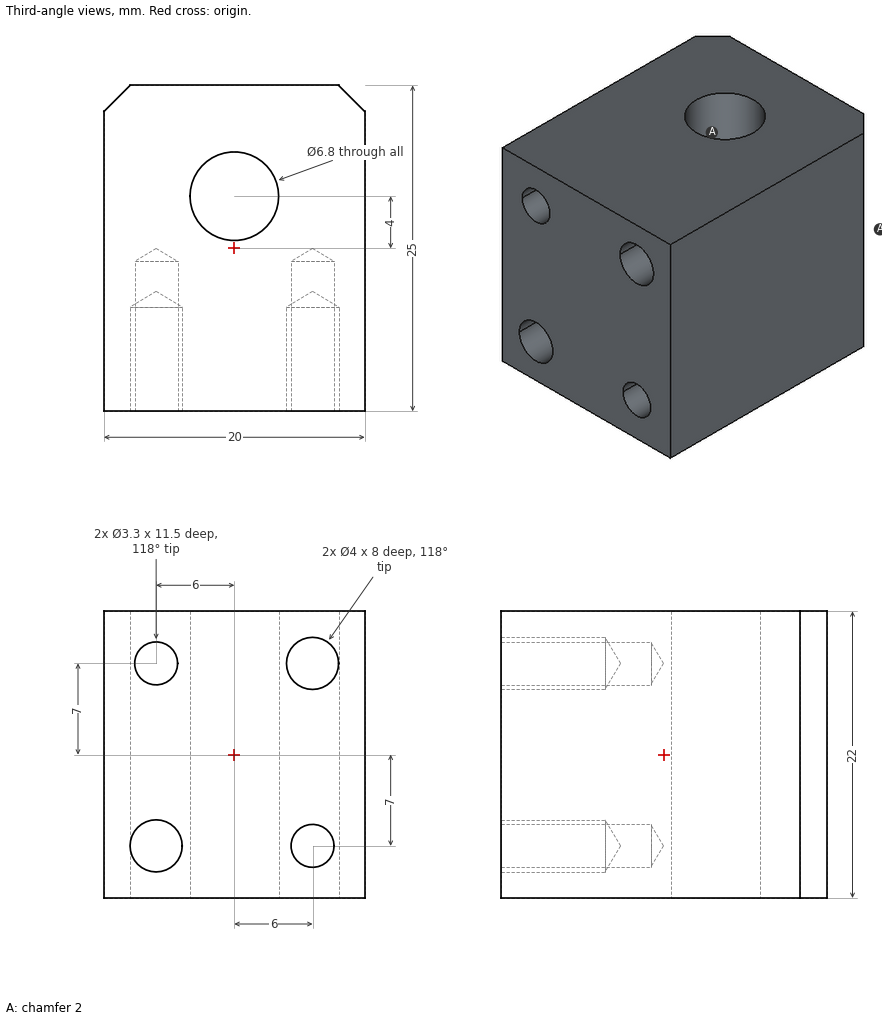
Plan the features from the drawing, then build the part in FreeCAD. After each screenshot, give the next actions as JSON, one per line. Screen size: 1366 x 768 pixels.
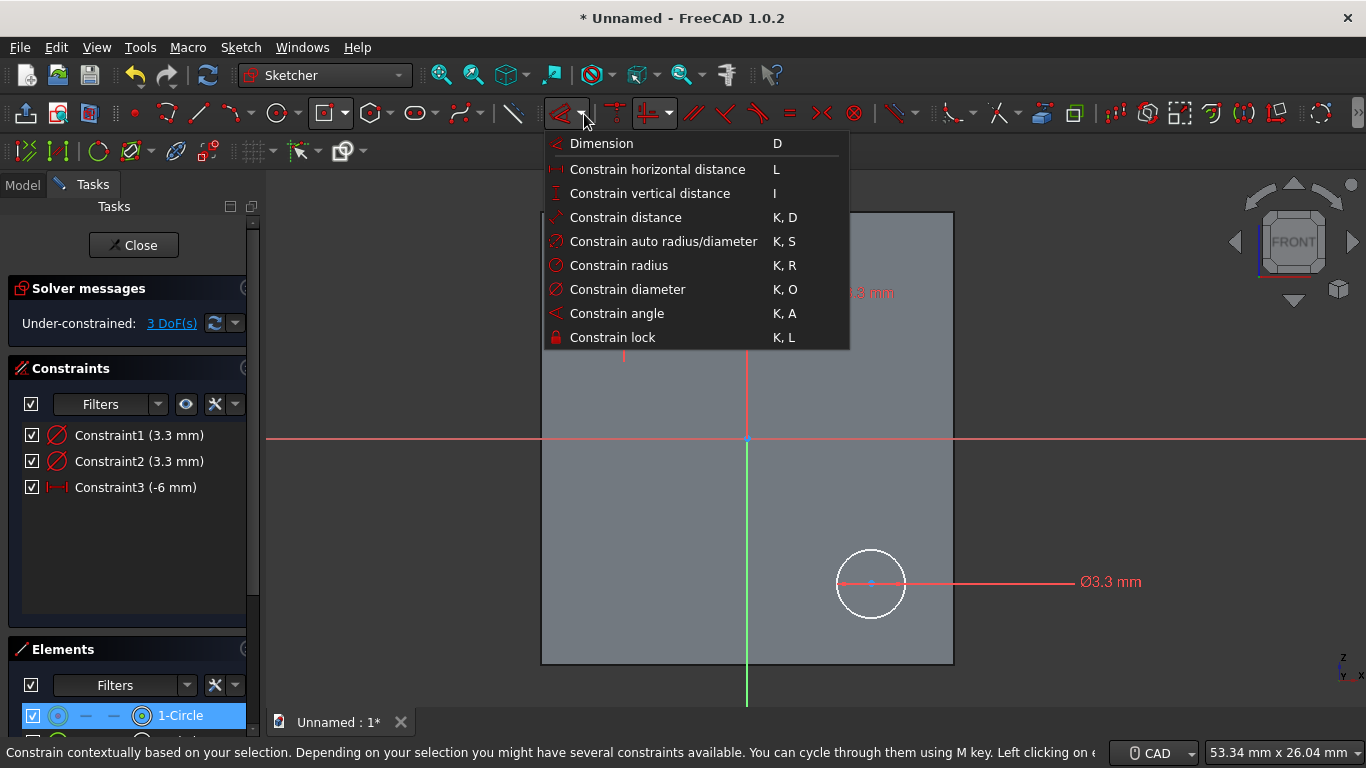
{"action": "left_click", "coordinate": [697, 193]}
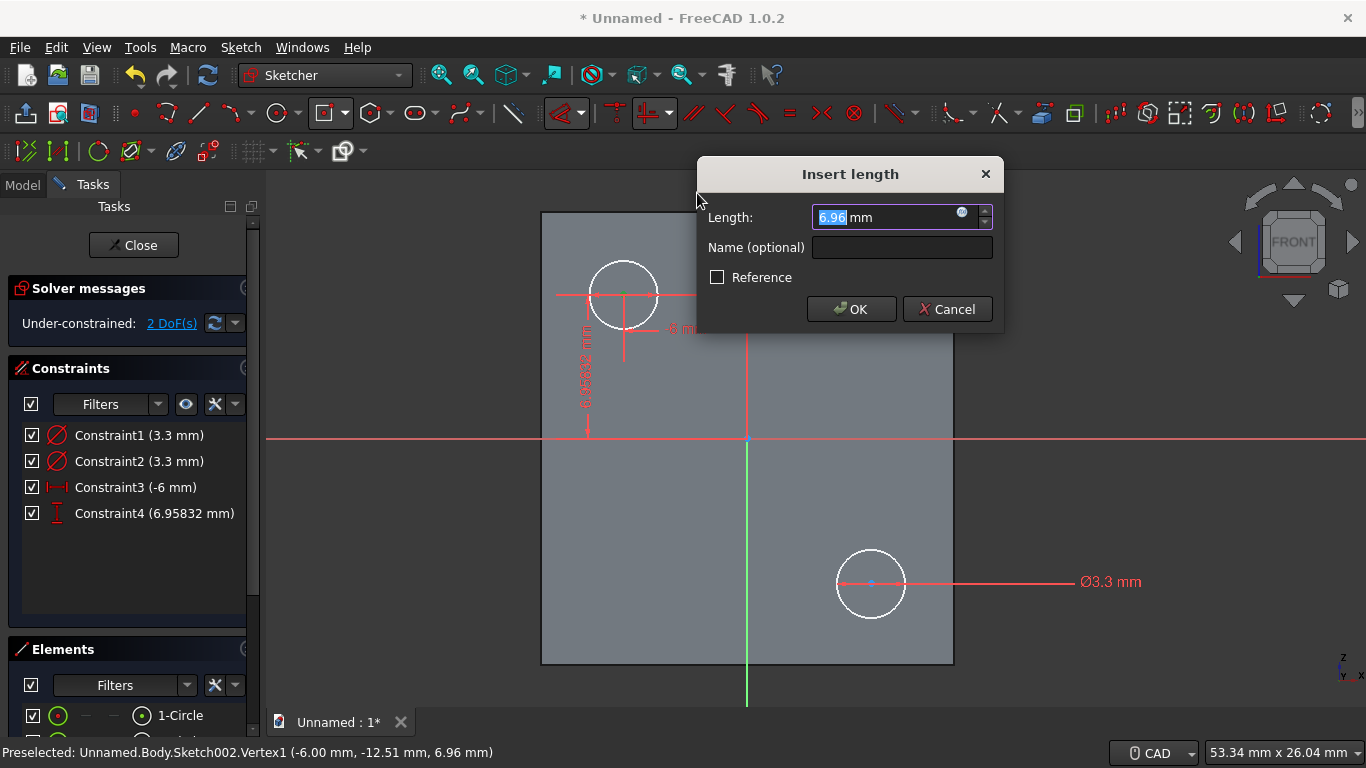
{"action": "type", "text": "7"}
{"action": "key", "text": "Return"}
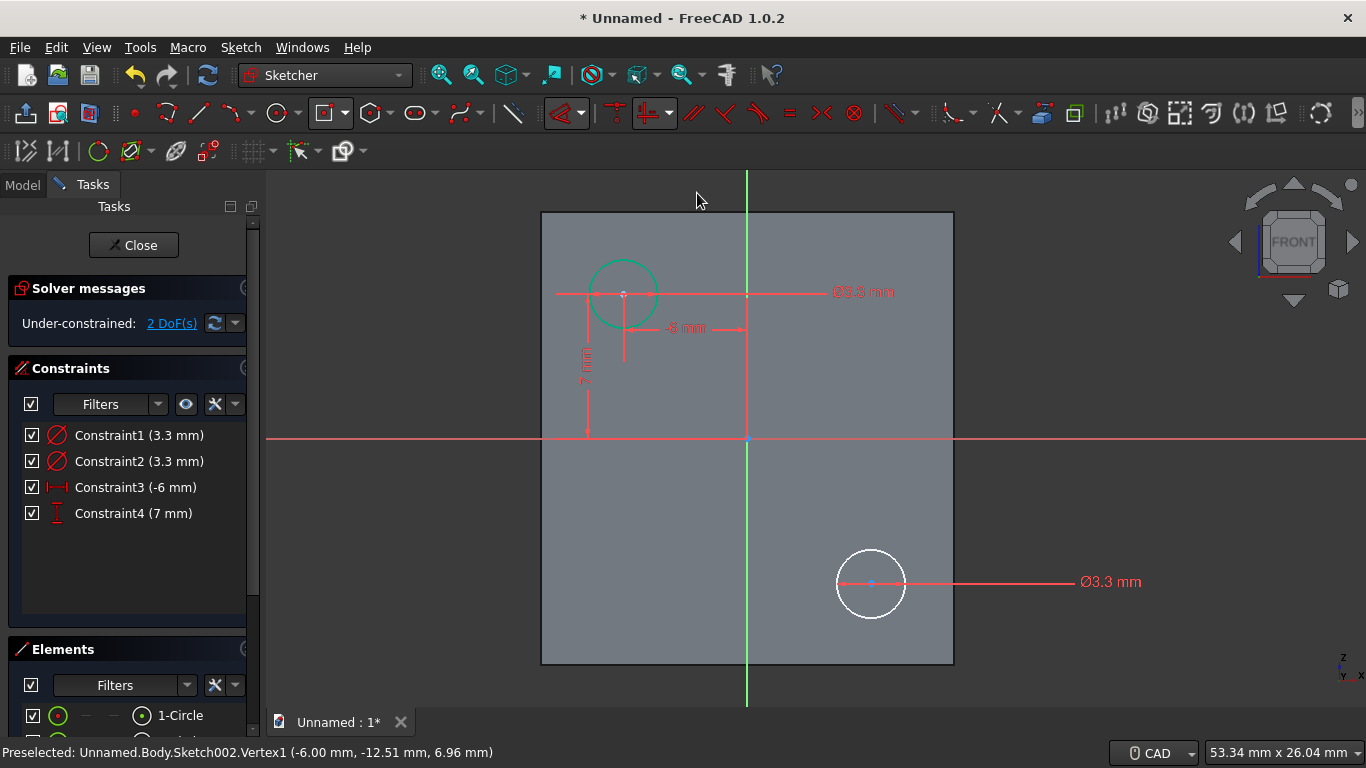
{"action": "left_click", "coordinate": [871, 584]}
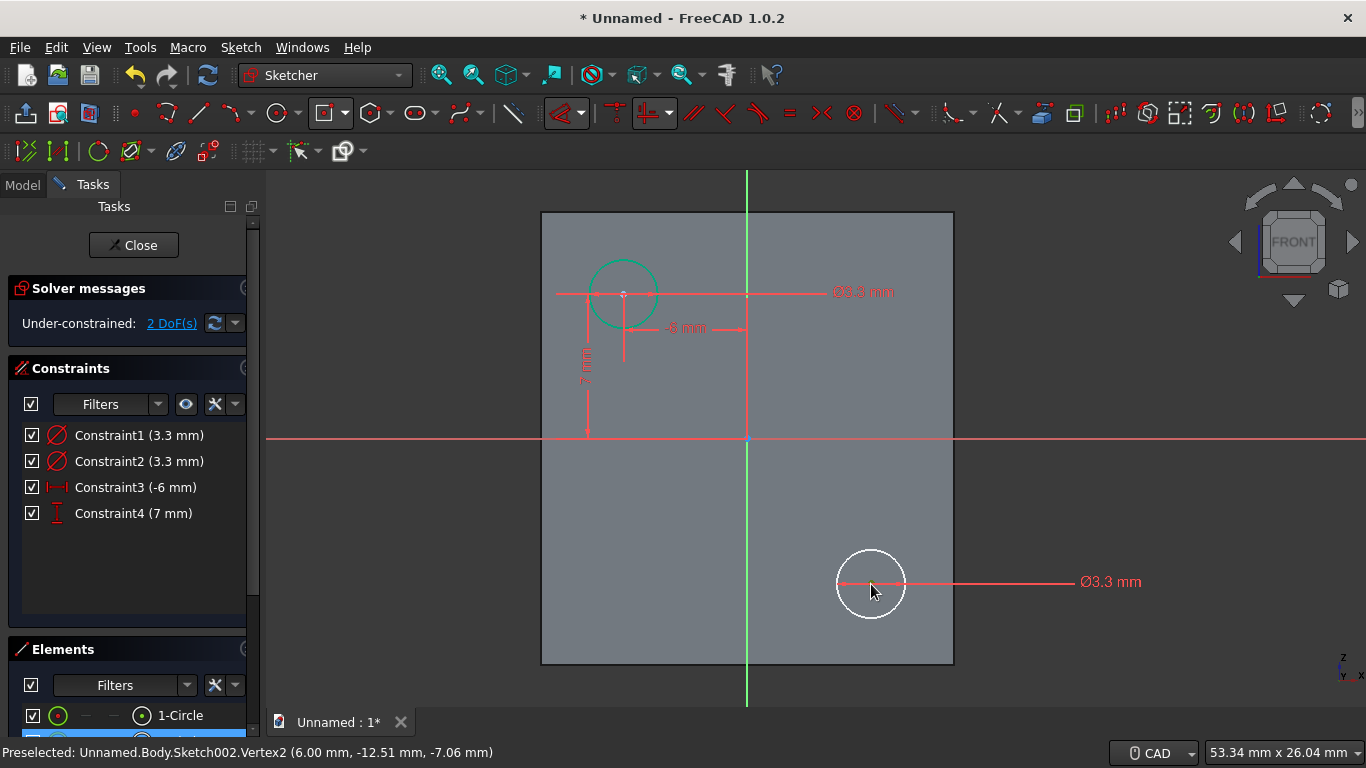
{"action": "key", "text": "l"}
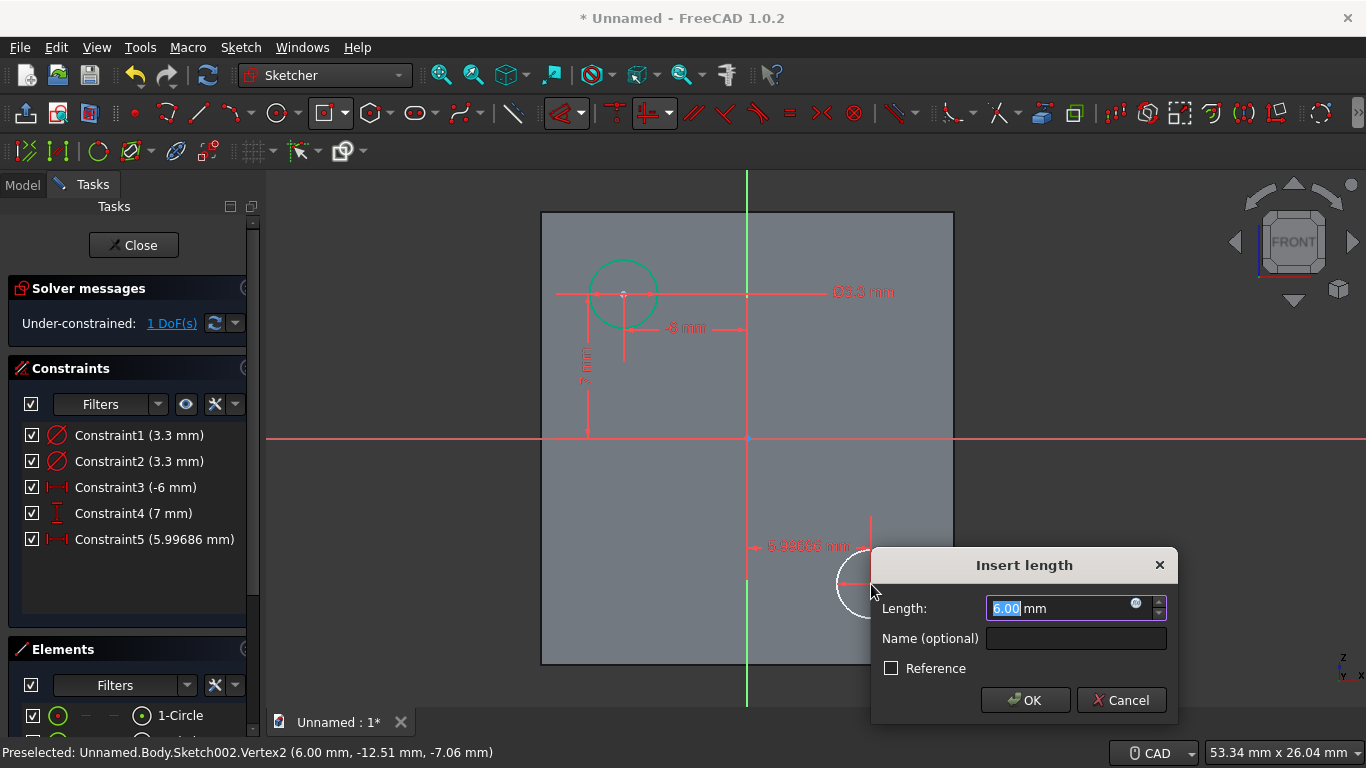
{"action": "type", "text": "6"}
{"action": "key", "text": "Return"}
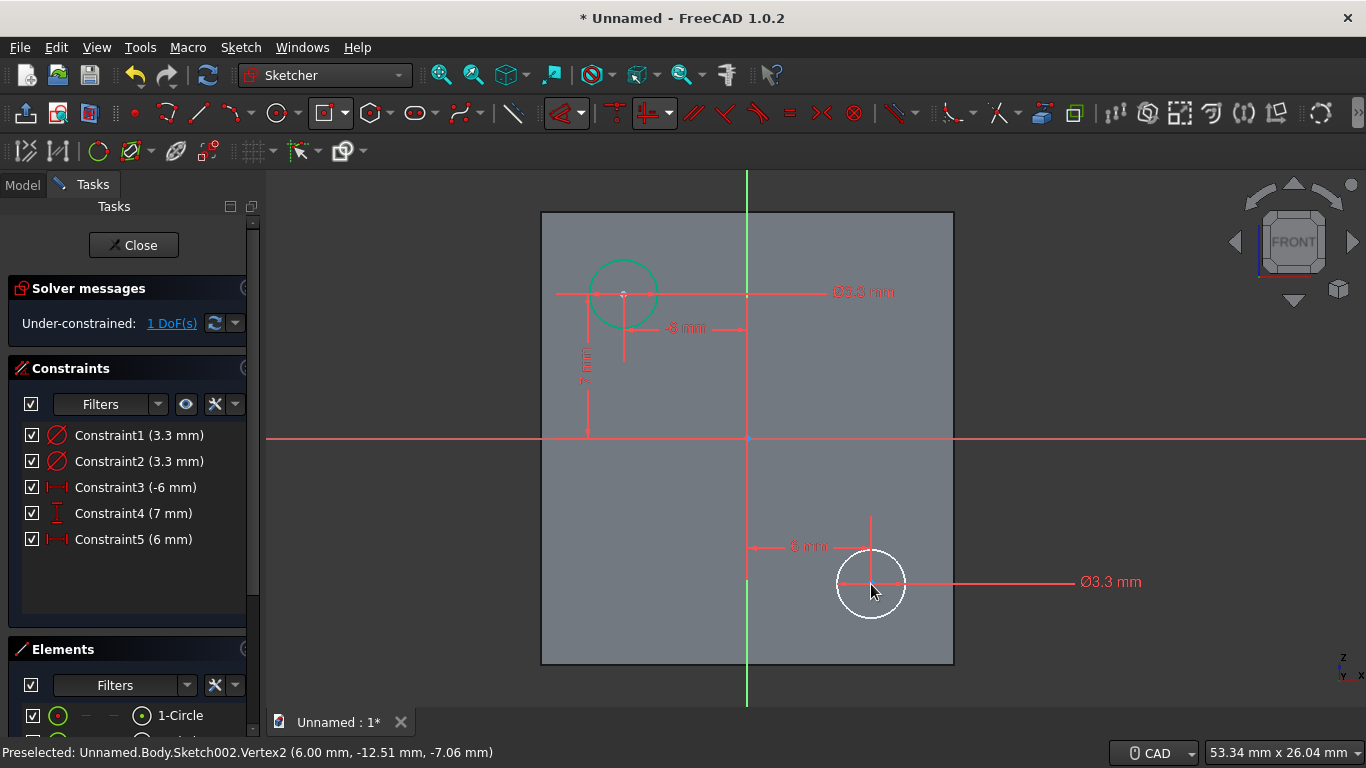
{"action": "left_click", "coordinate": [871, 584]}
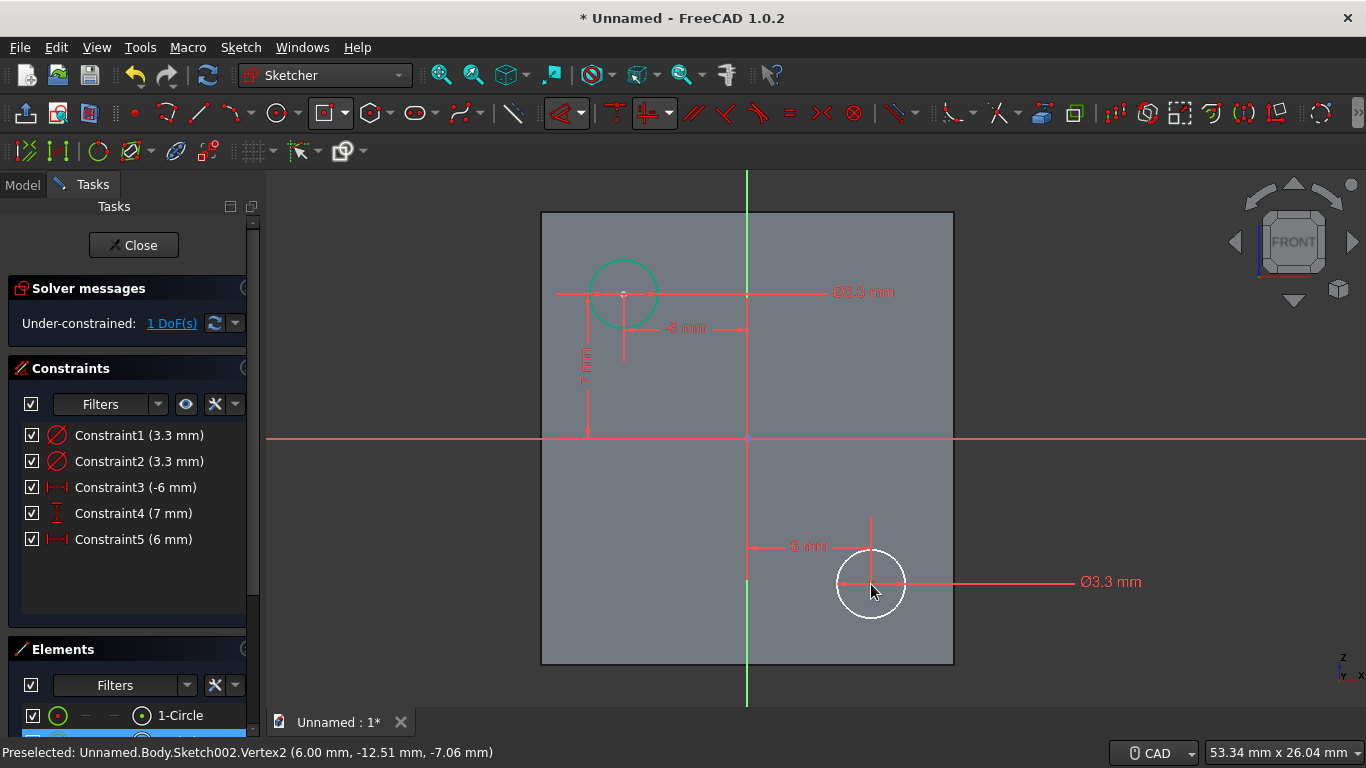
{"action": "left_click", "coordinate": [584, 114]}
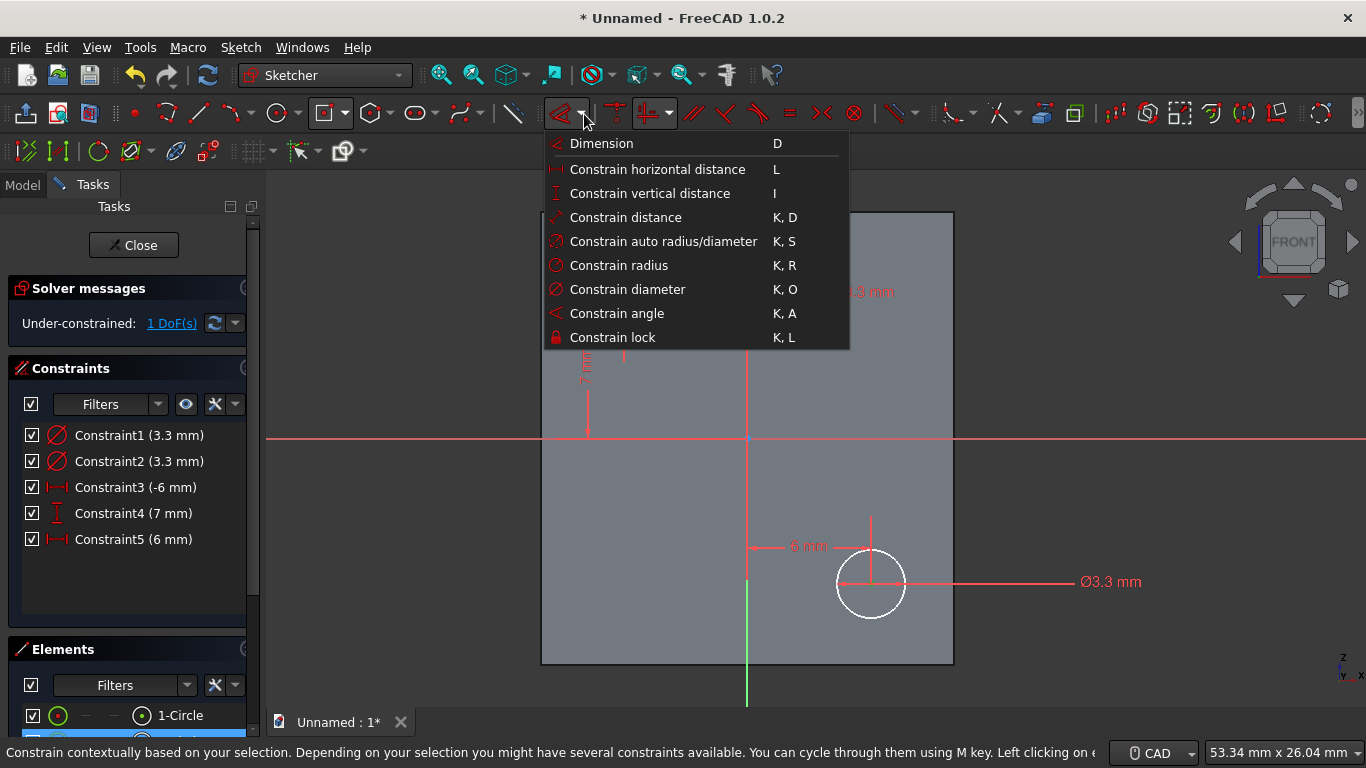
{"action": "left_click", "coordinate": [697, 193]}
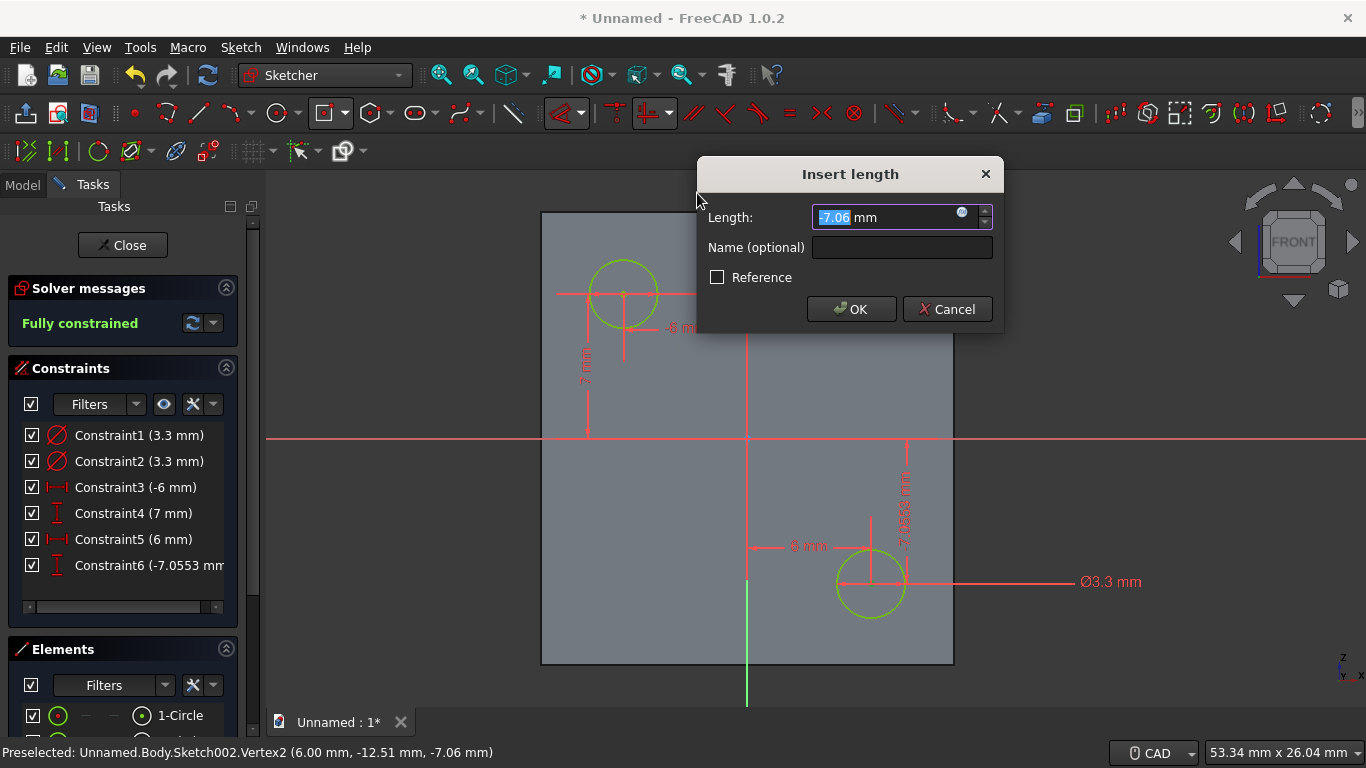
{"action": "type", "text": "-7"}
{"action": "key", "text": "Return"}